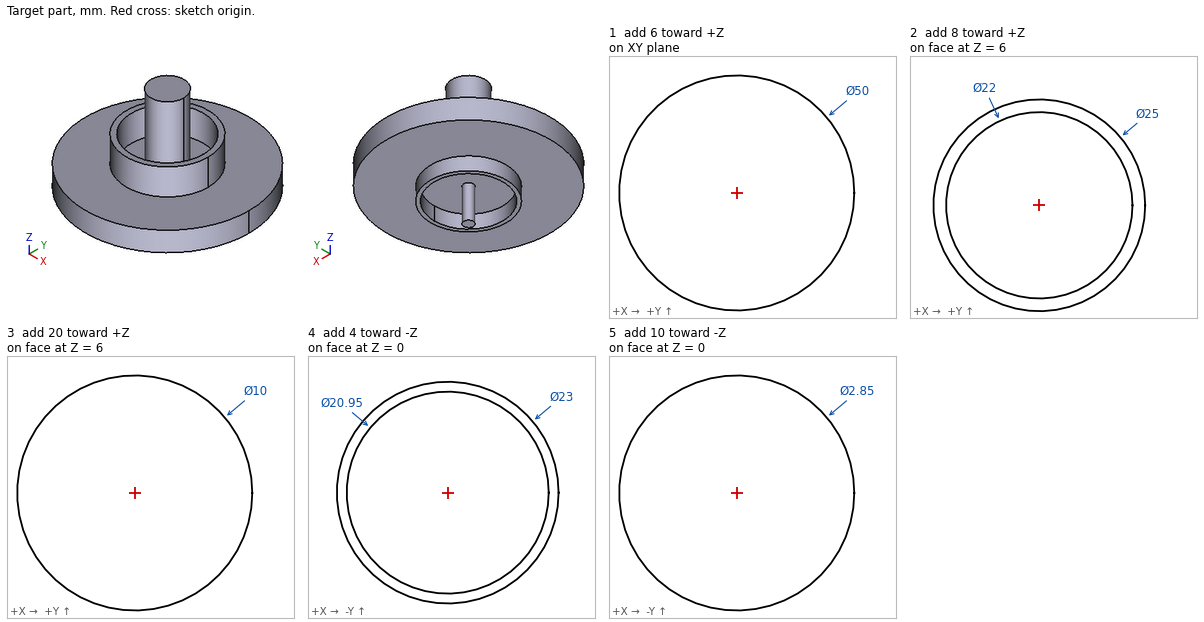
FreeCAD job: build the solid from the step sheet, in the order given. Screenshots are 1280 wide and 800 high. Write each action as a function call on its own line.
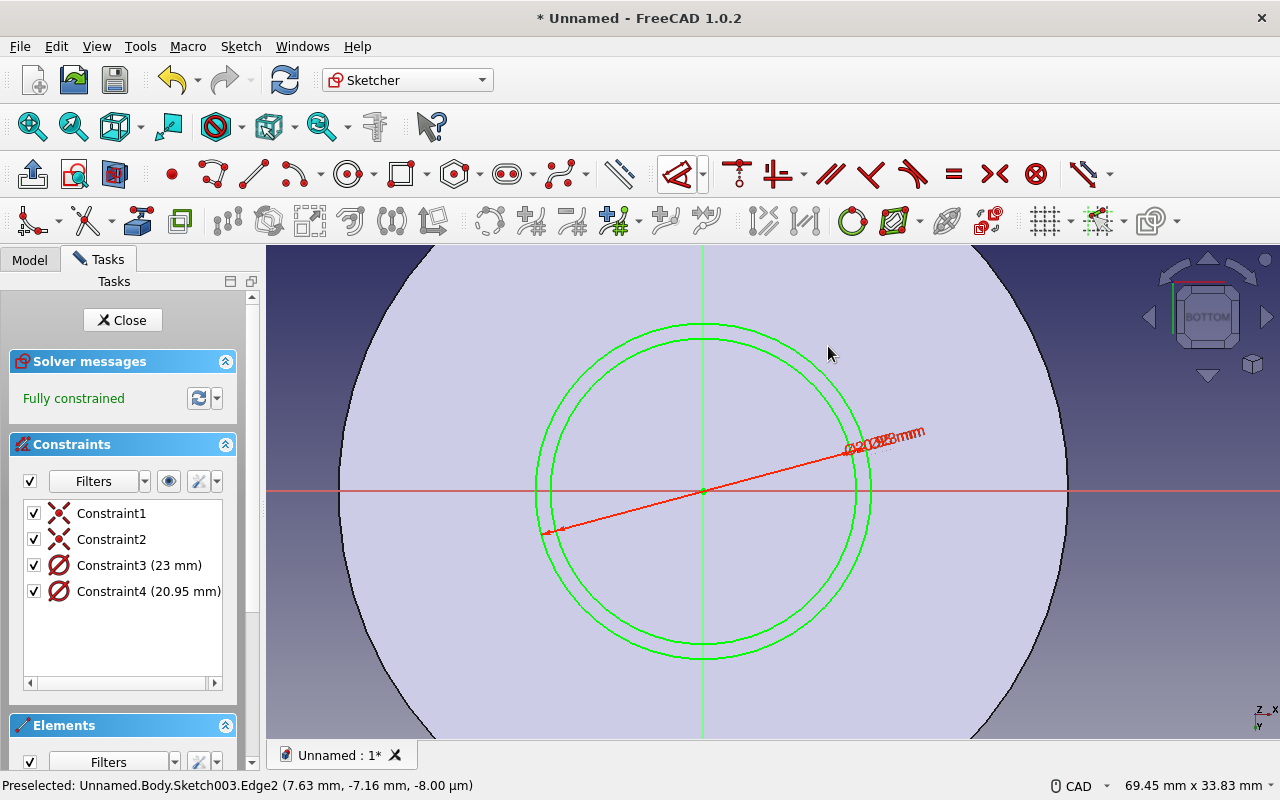
click(123, 320)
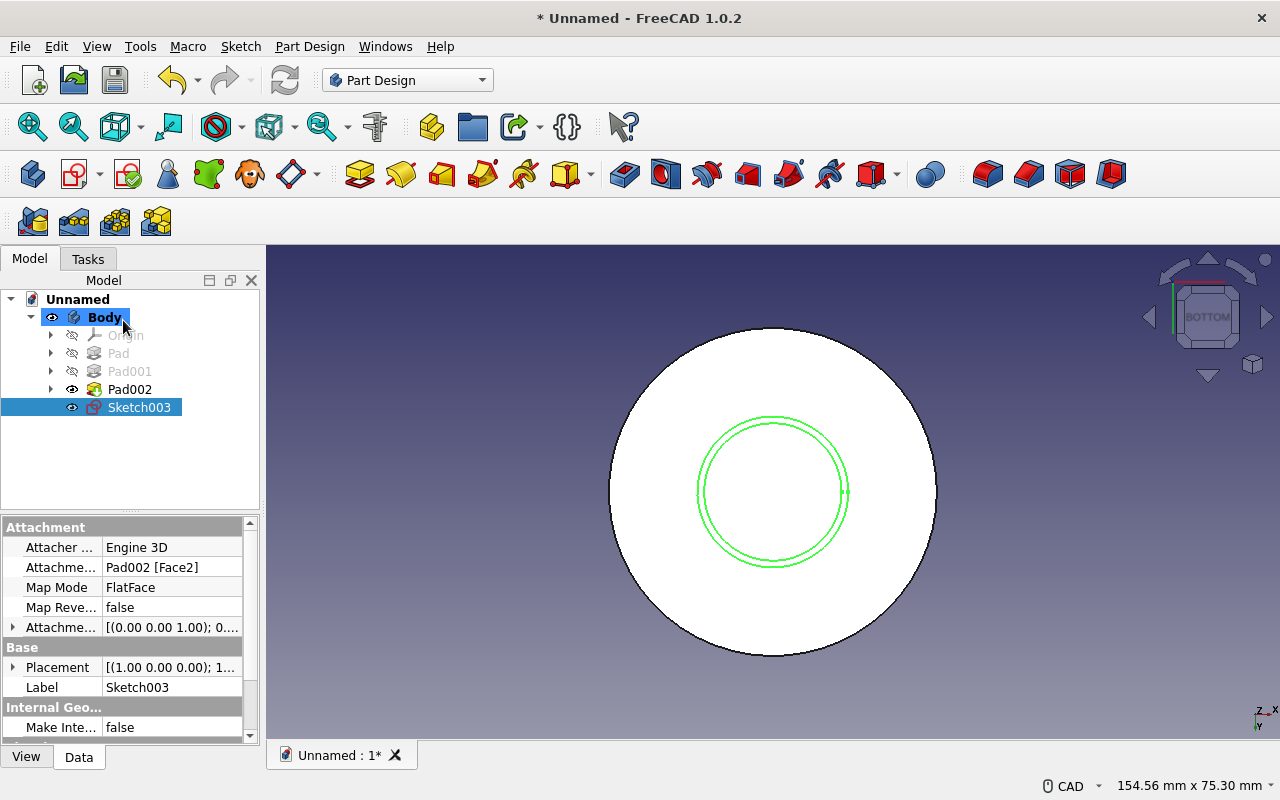
click(360, 174)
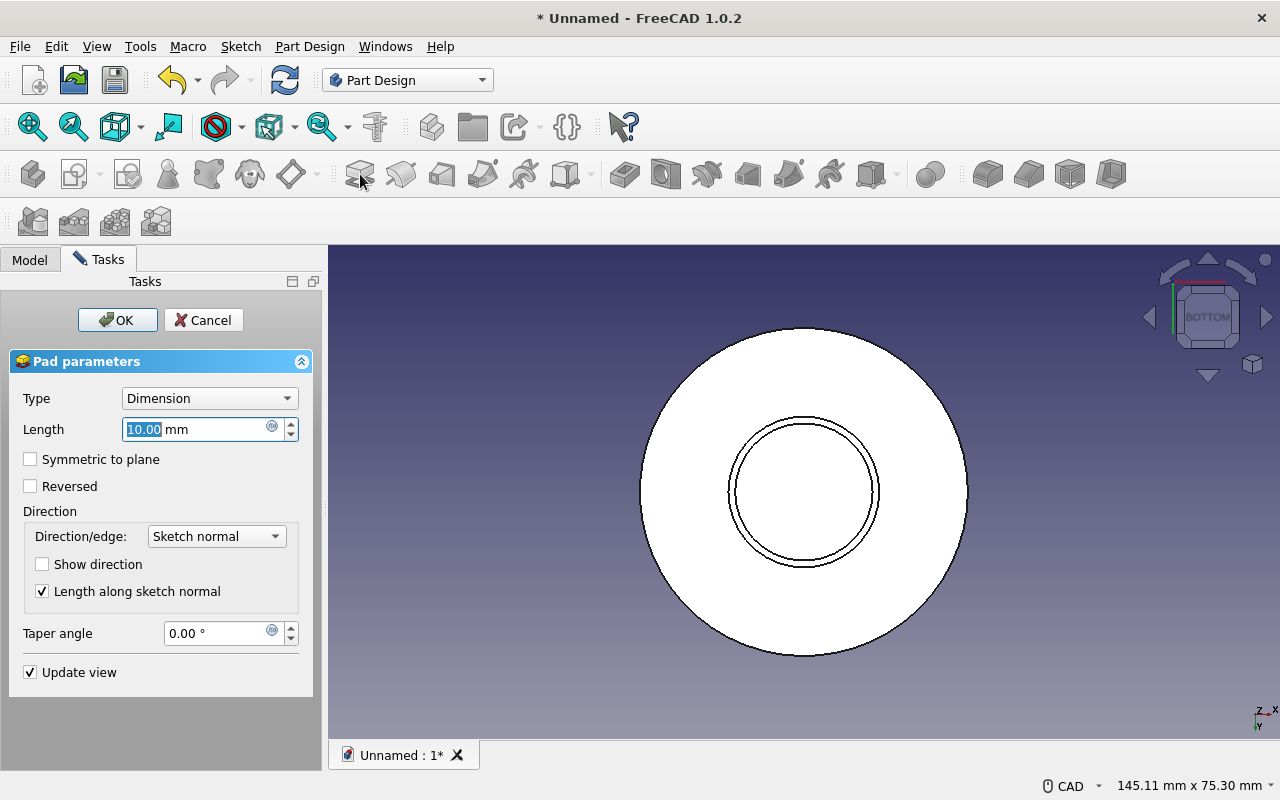
text(4)
key(Tab)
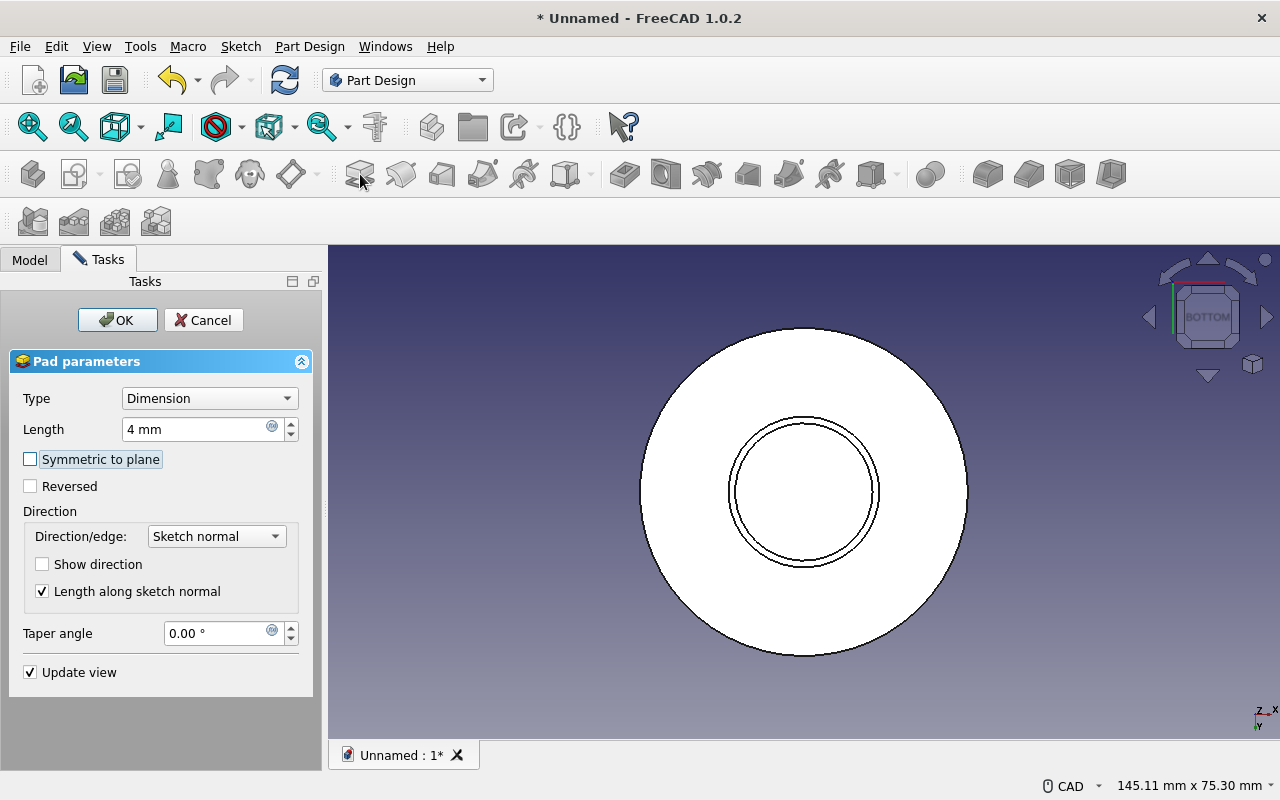
click(118, 320)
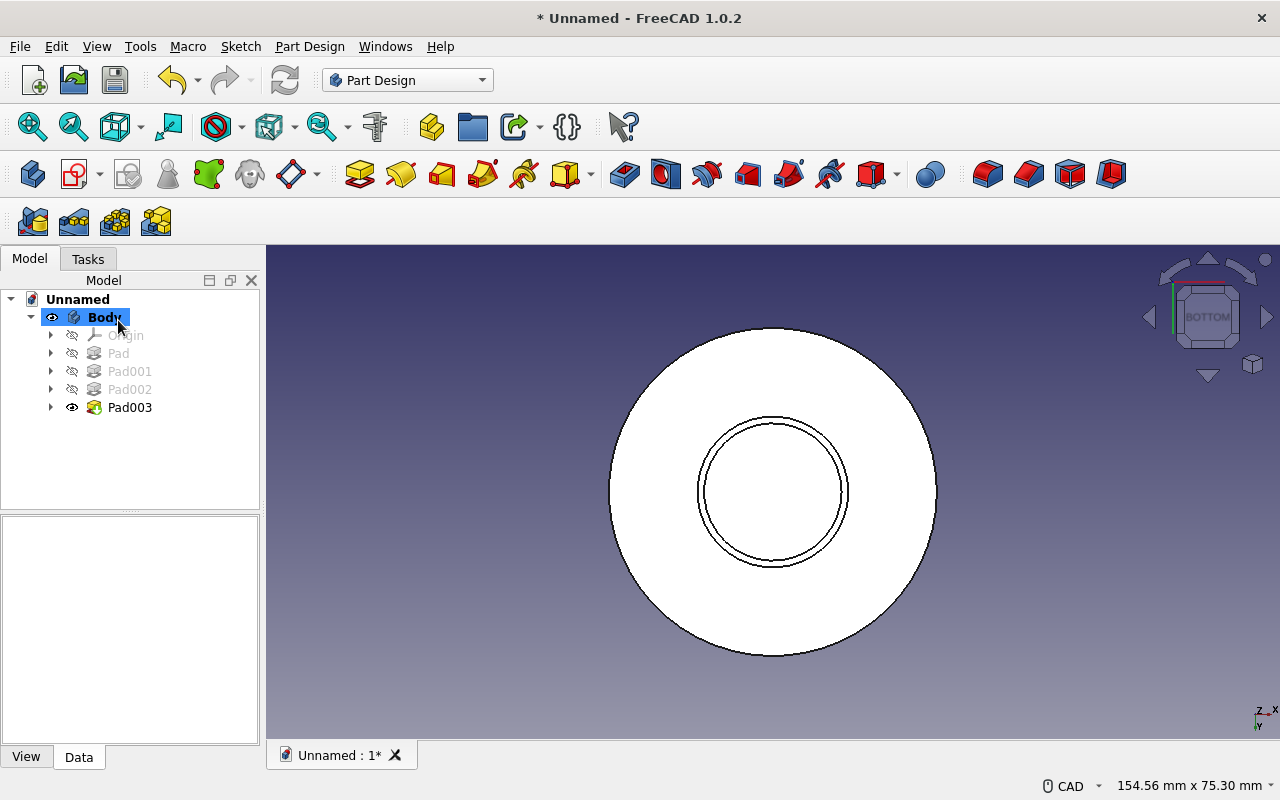
click(867, 397)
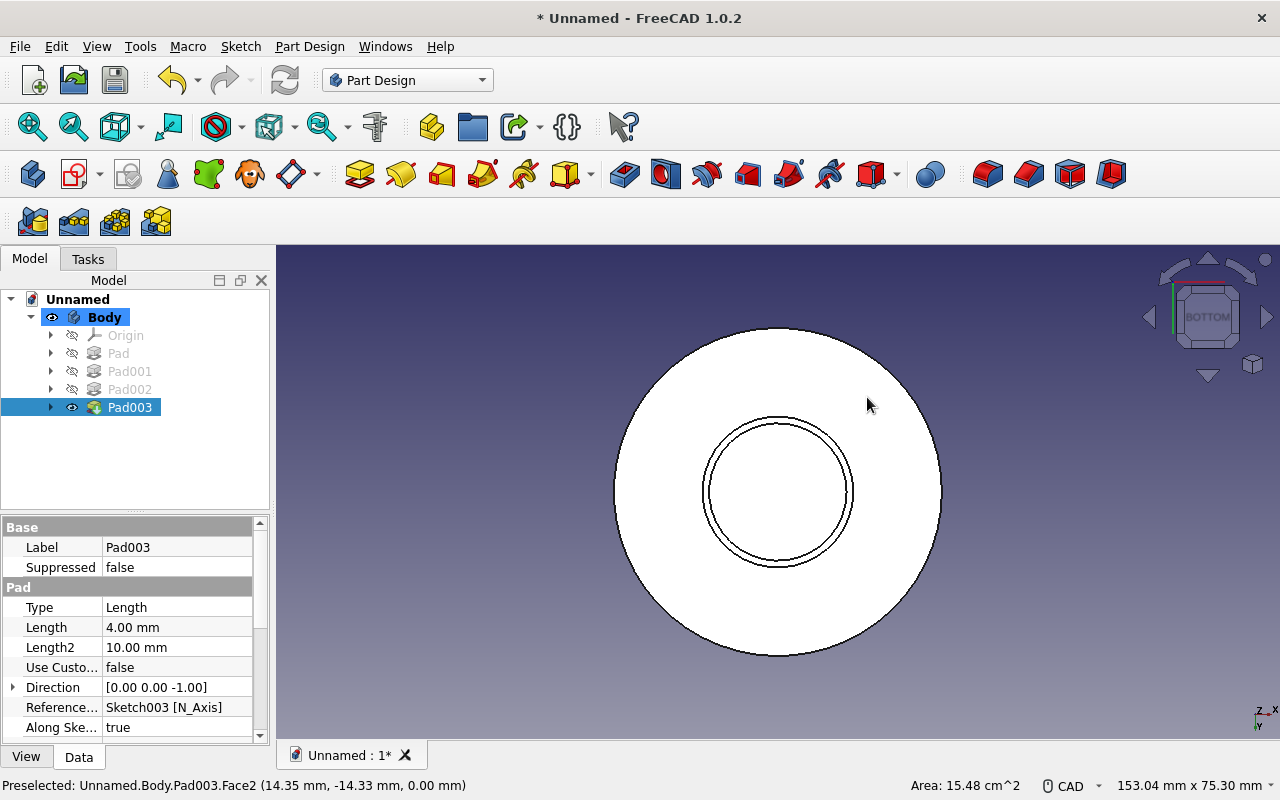
click(74, 174)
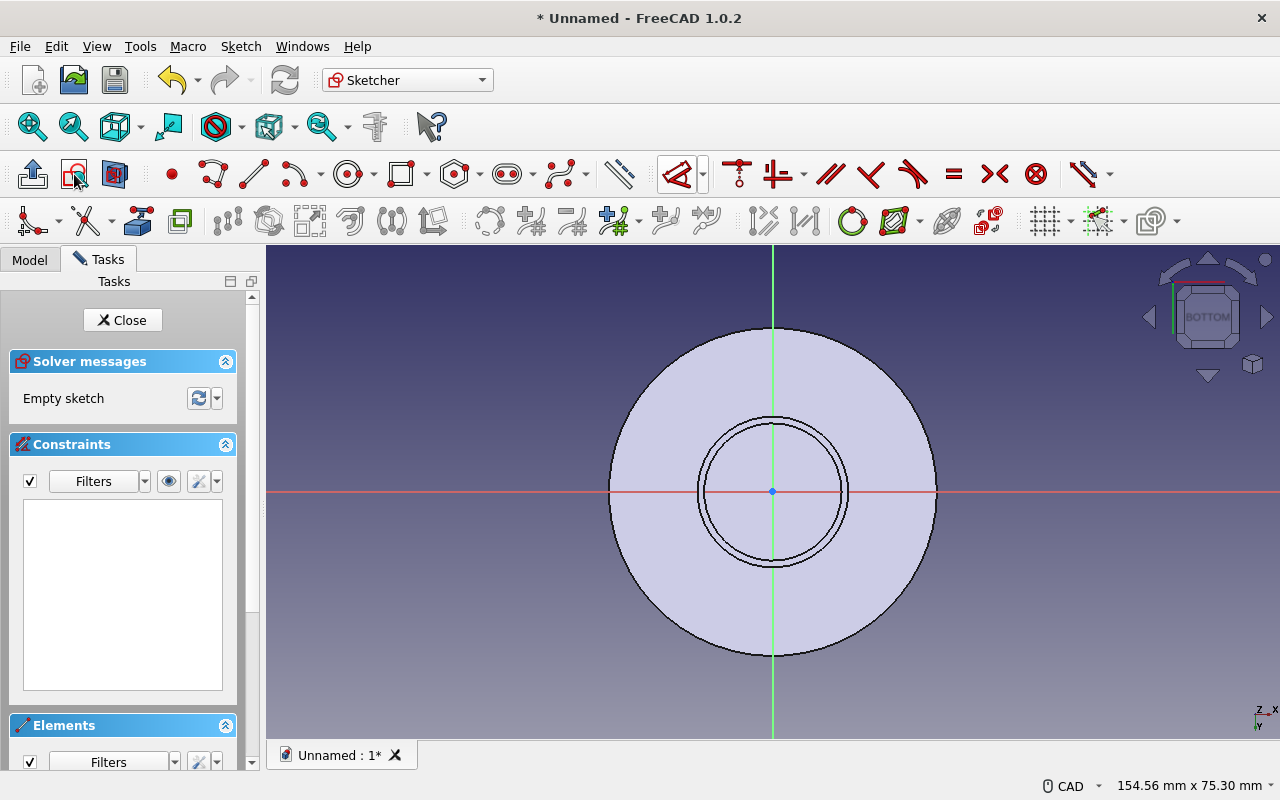
click(115, 174)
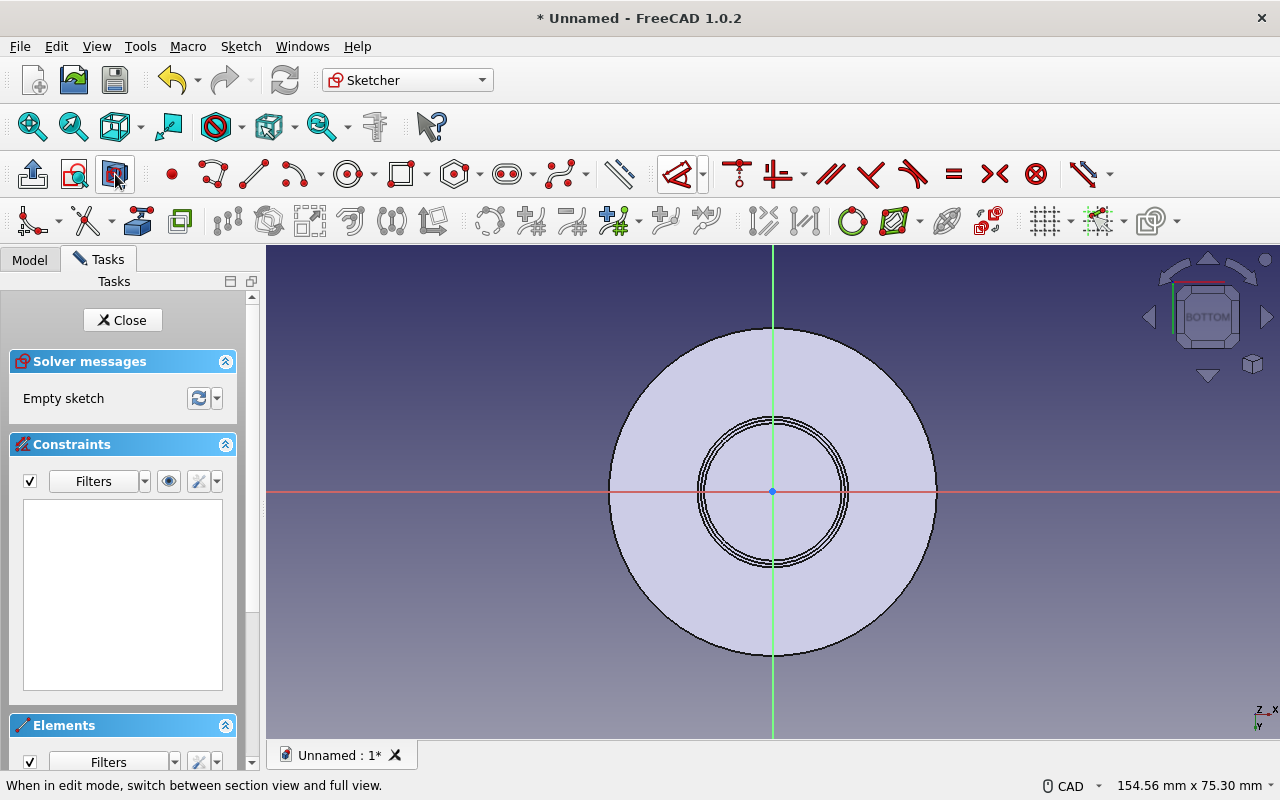
scroll(777, 492, up, 14)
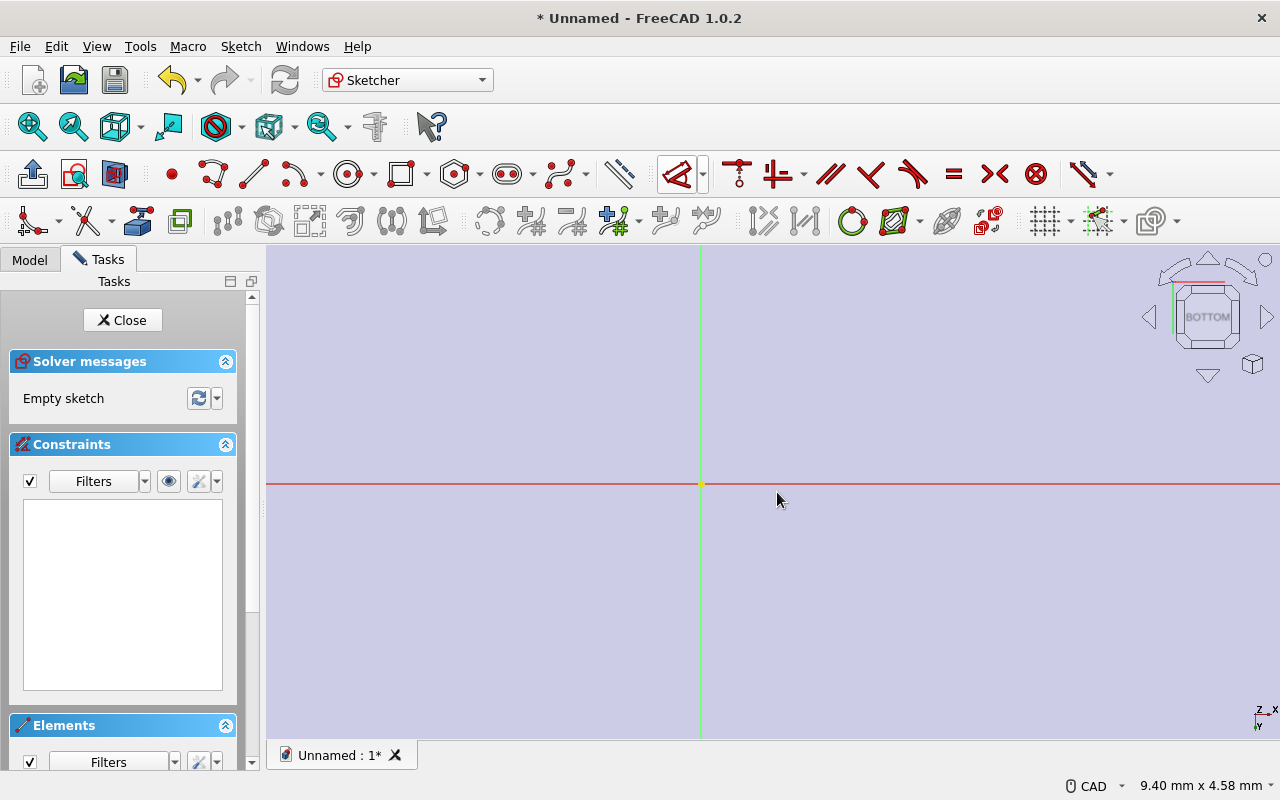
click(348, 174)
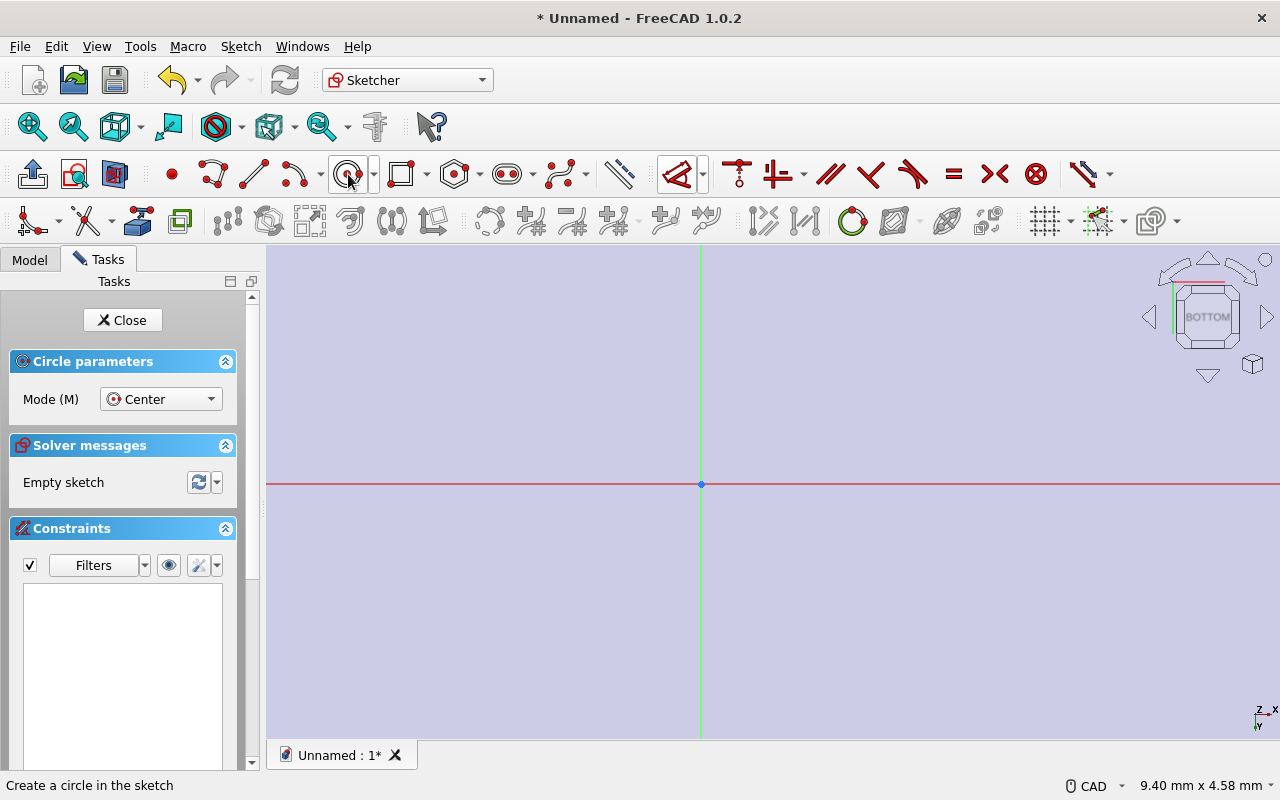
click(701, 484)
click(810, 376)
key(Escape)